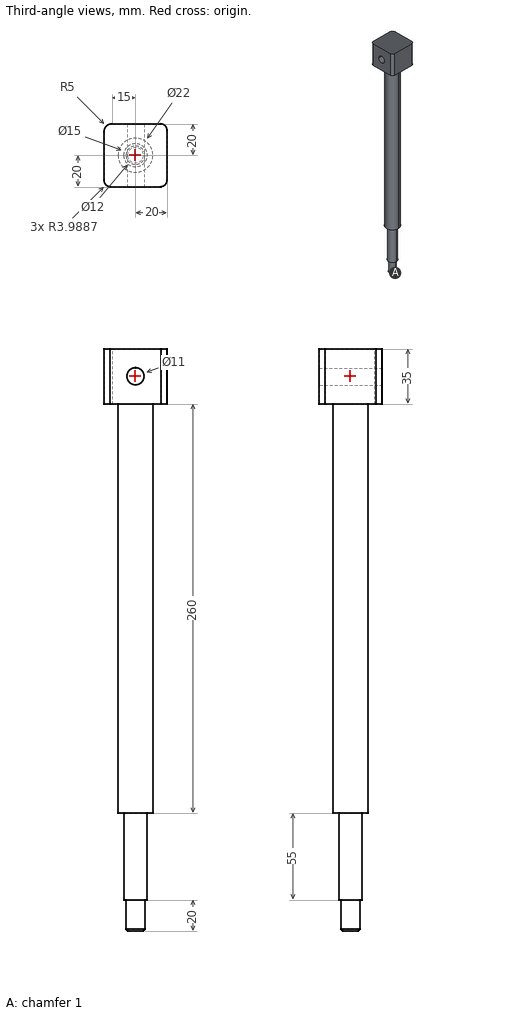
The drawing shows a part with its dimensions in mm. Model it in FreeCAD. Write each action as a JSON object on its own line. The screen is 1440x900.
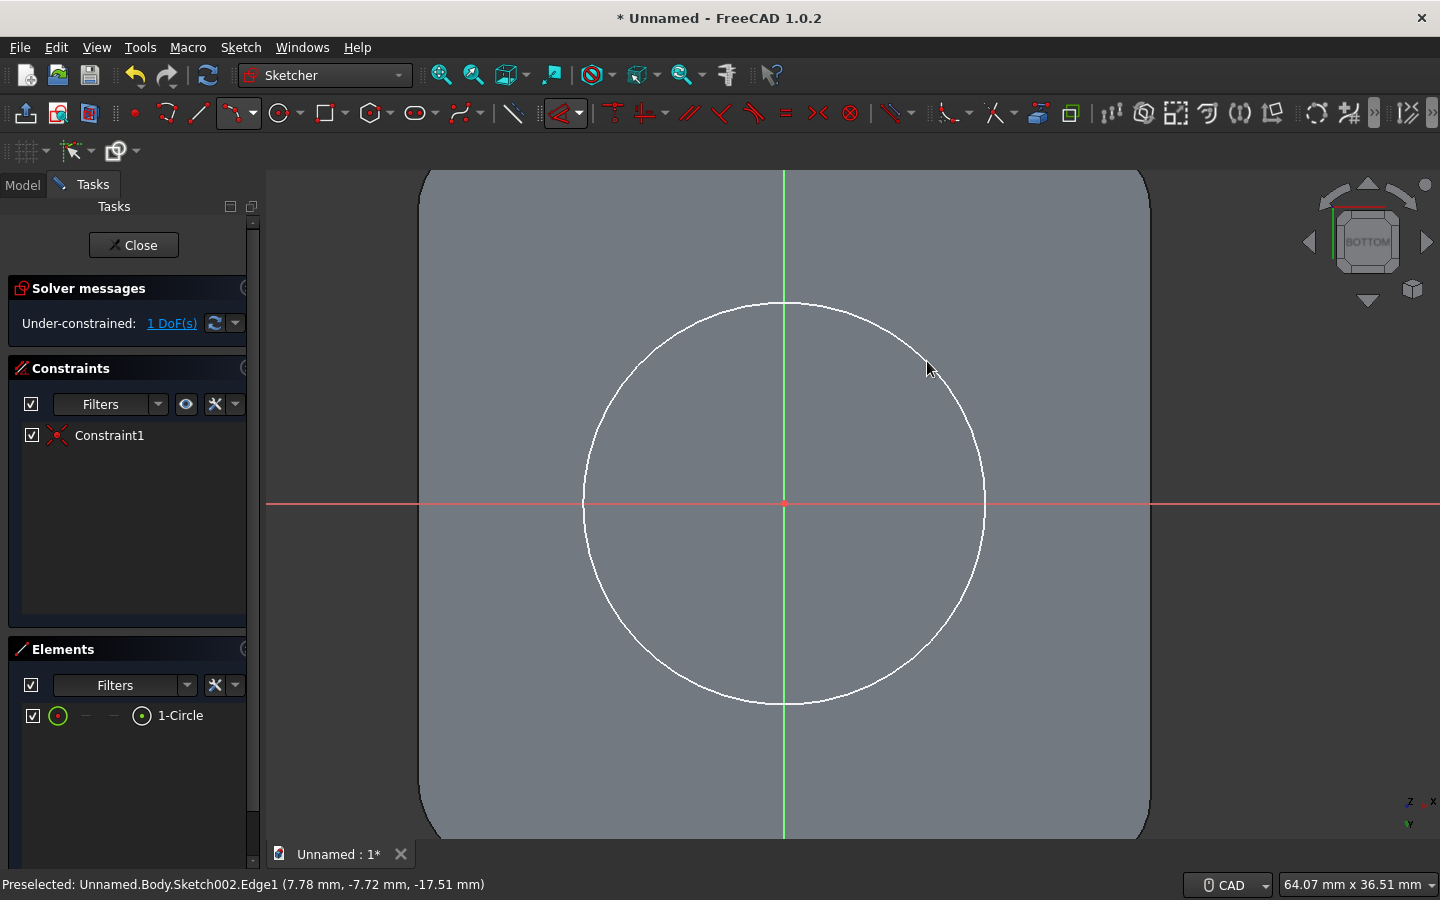
{"action": "left_click", "coordinate": [926, 361]}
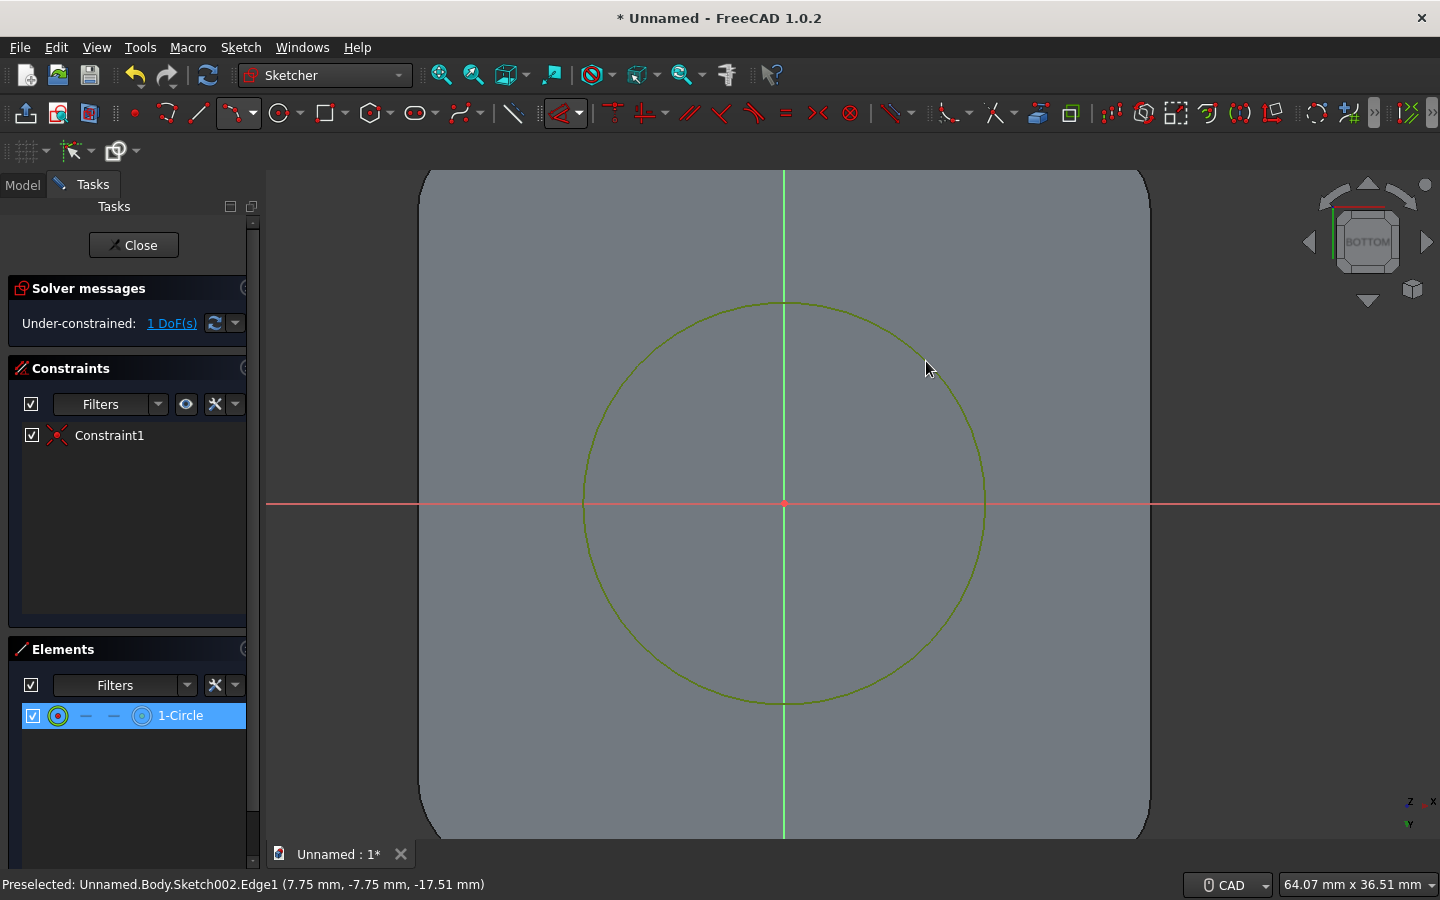
{"action": "left_click", "coordinate": [582, 114]}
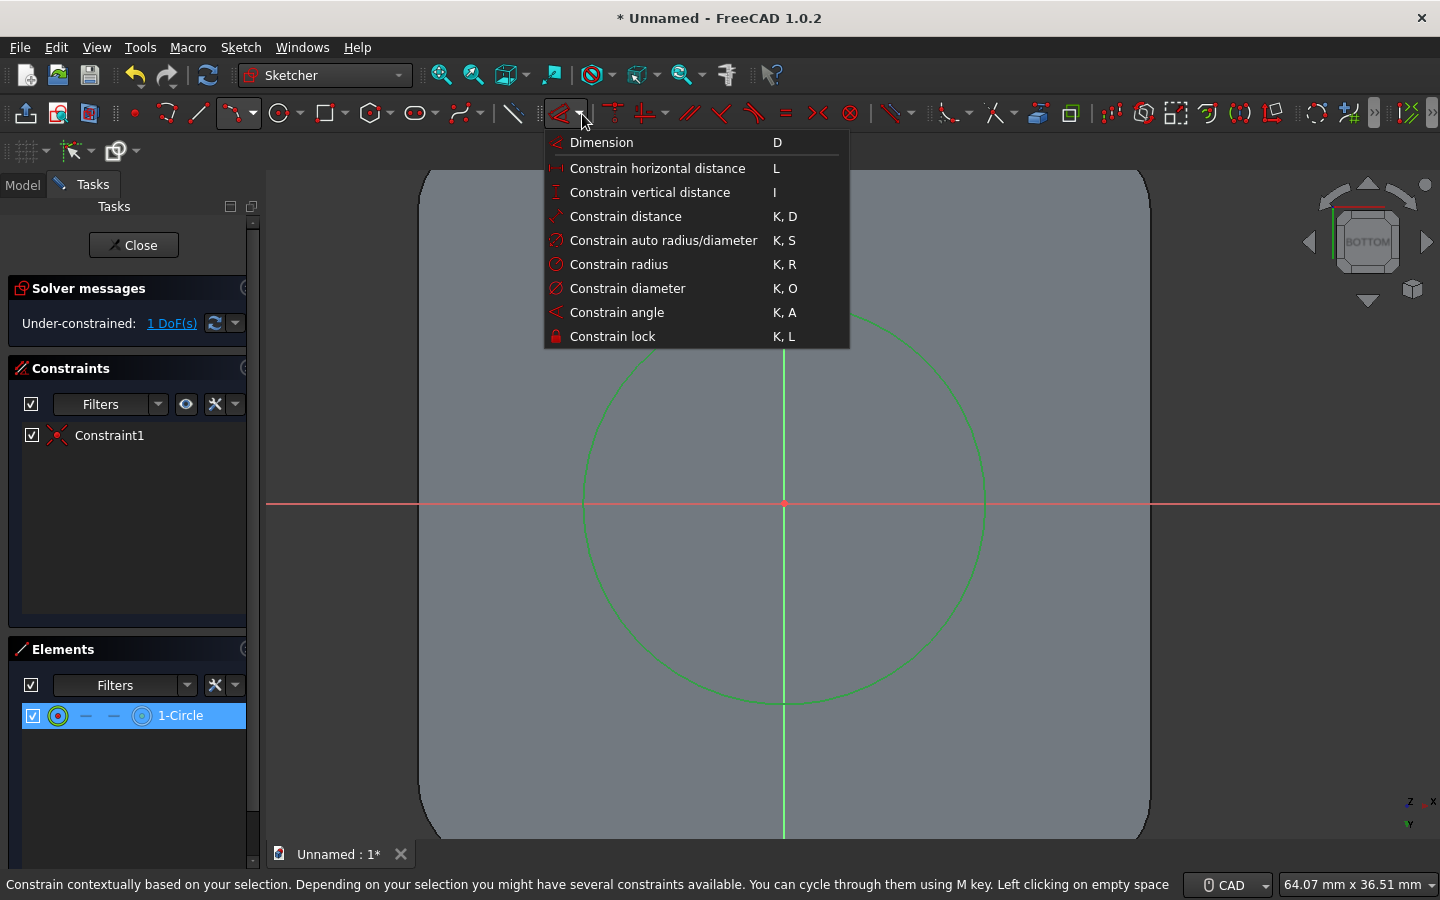
{"action": "left_click", "coordinate": [697, 288]}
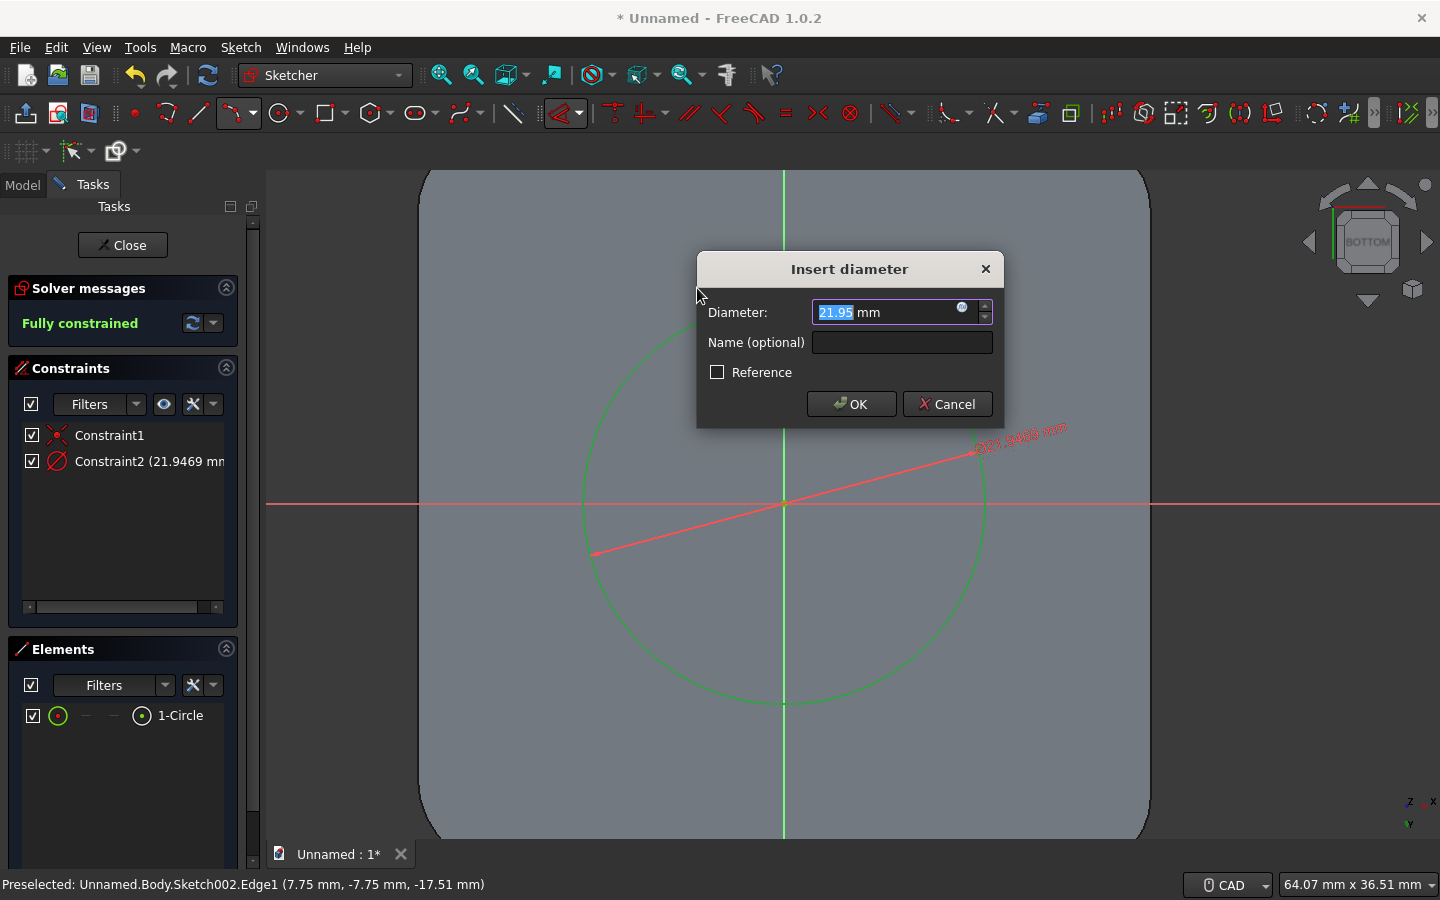
{"action": "type", "text": "22"}
{"action": "key", "text": "Return"}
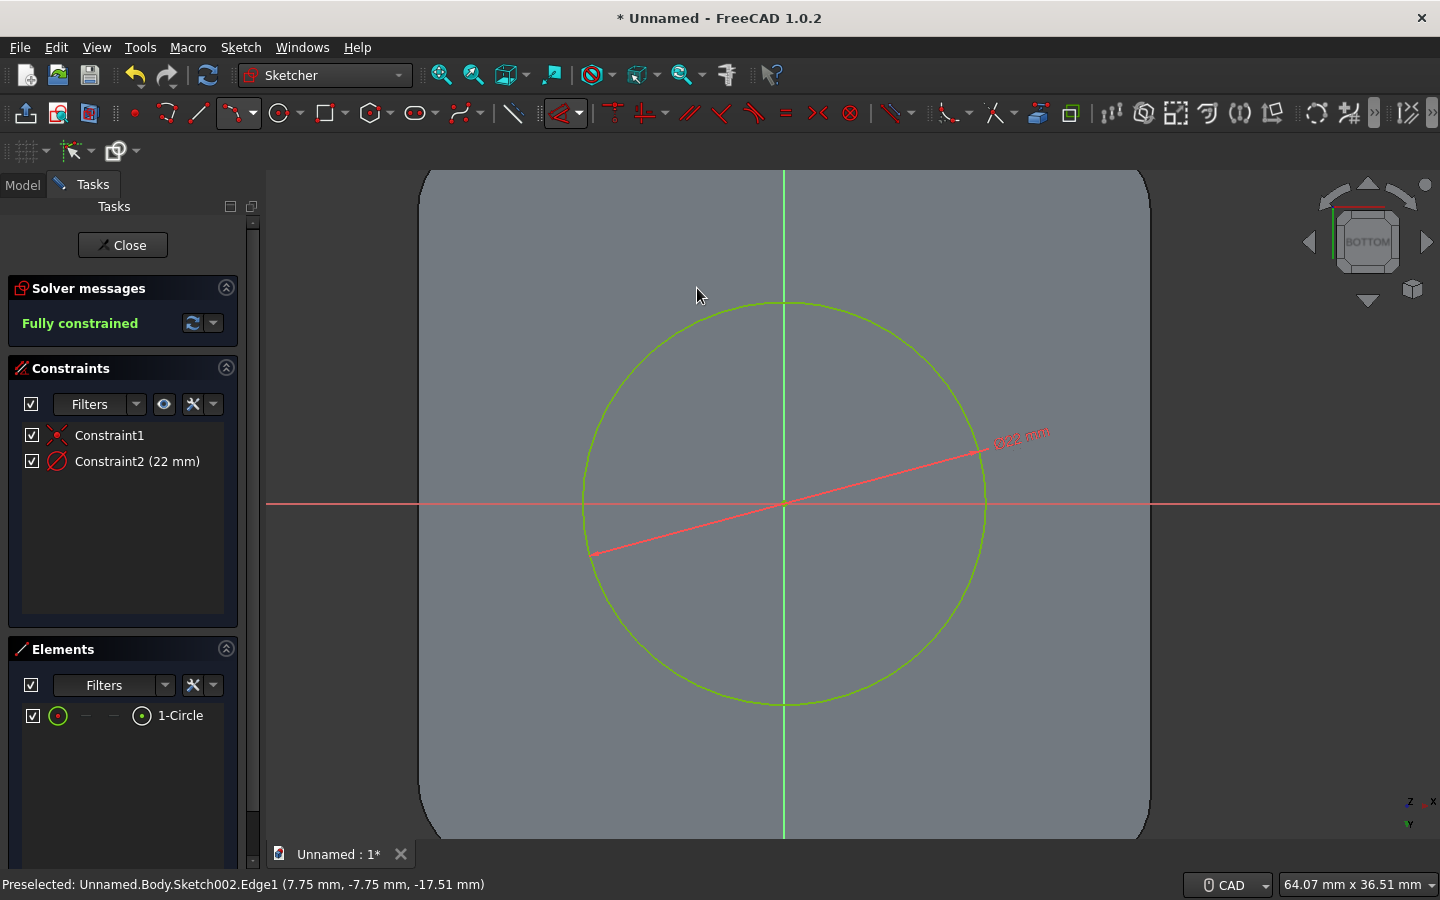
{"action": "left_click", "coordinate": [123, 245]}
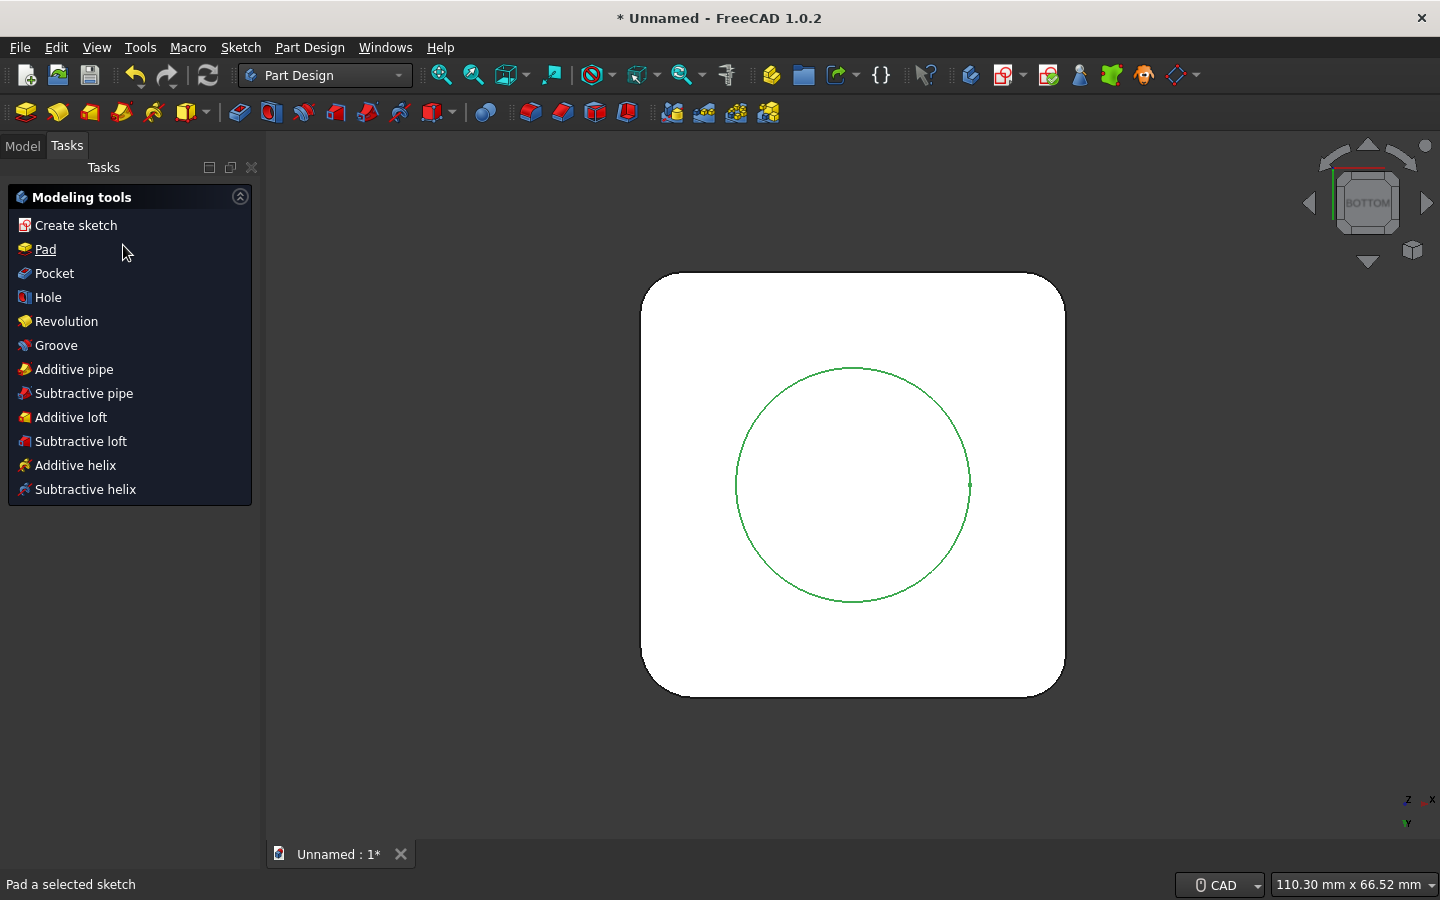
{"action": "left_click", "coordinate": [26, 112]}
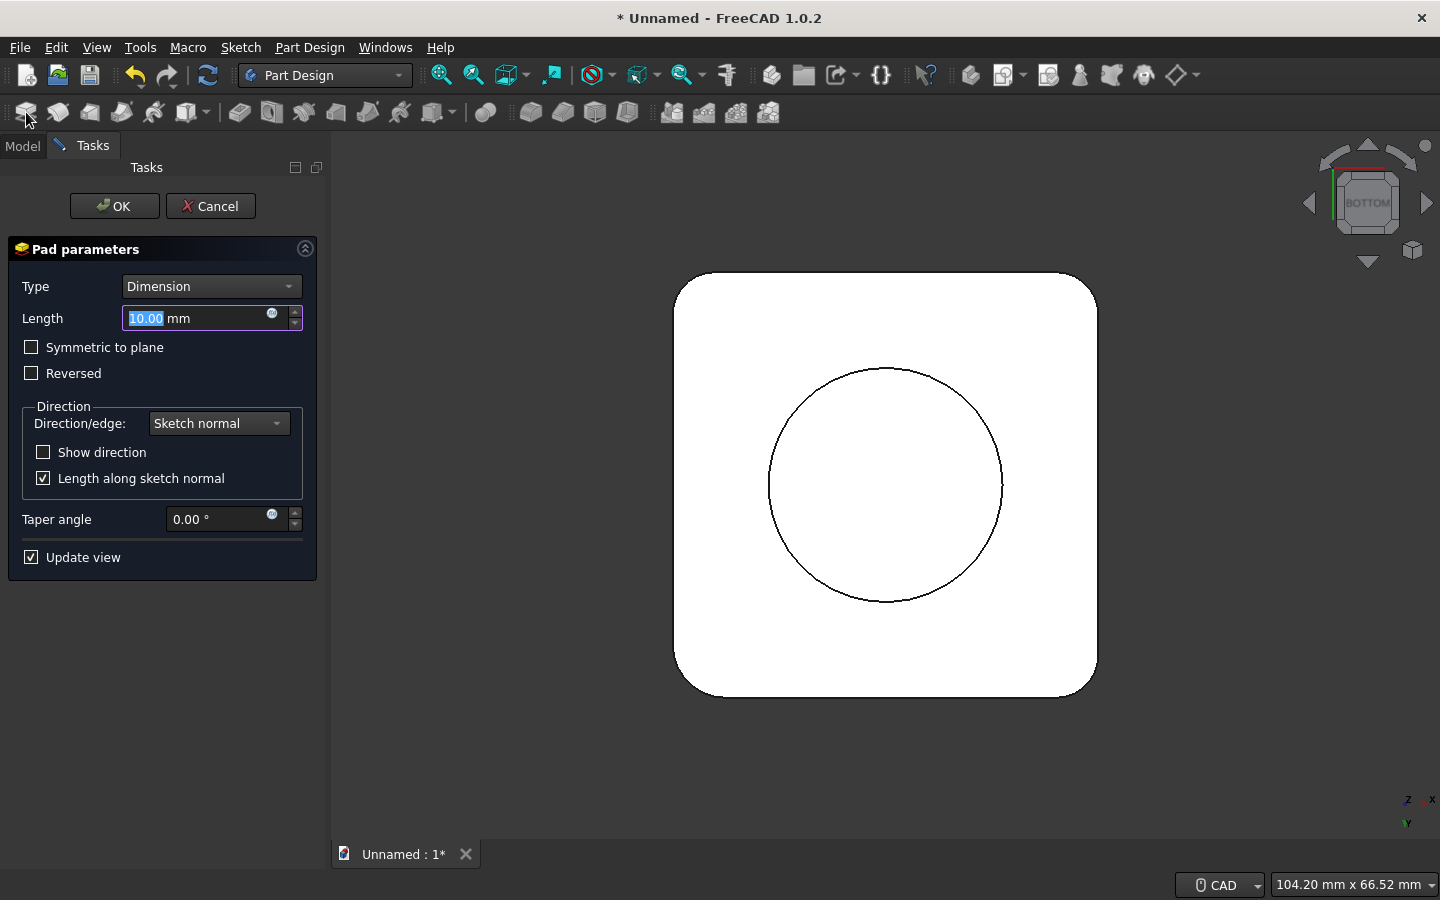
{"action": "type", "text": "260"}
{"action": "key", "text": "Tab"}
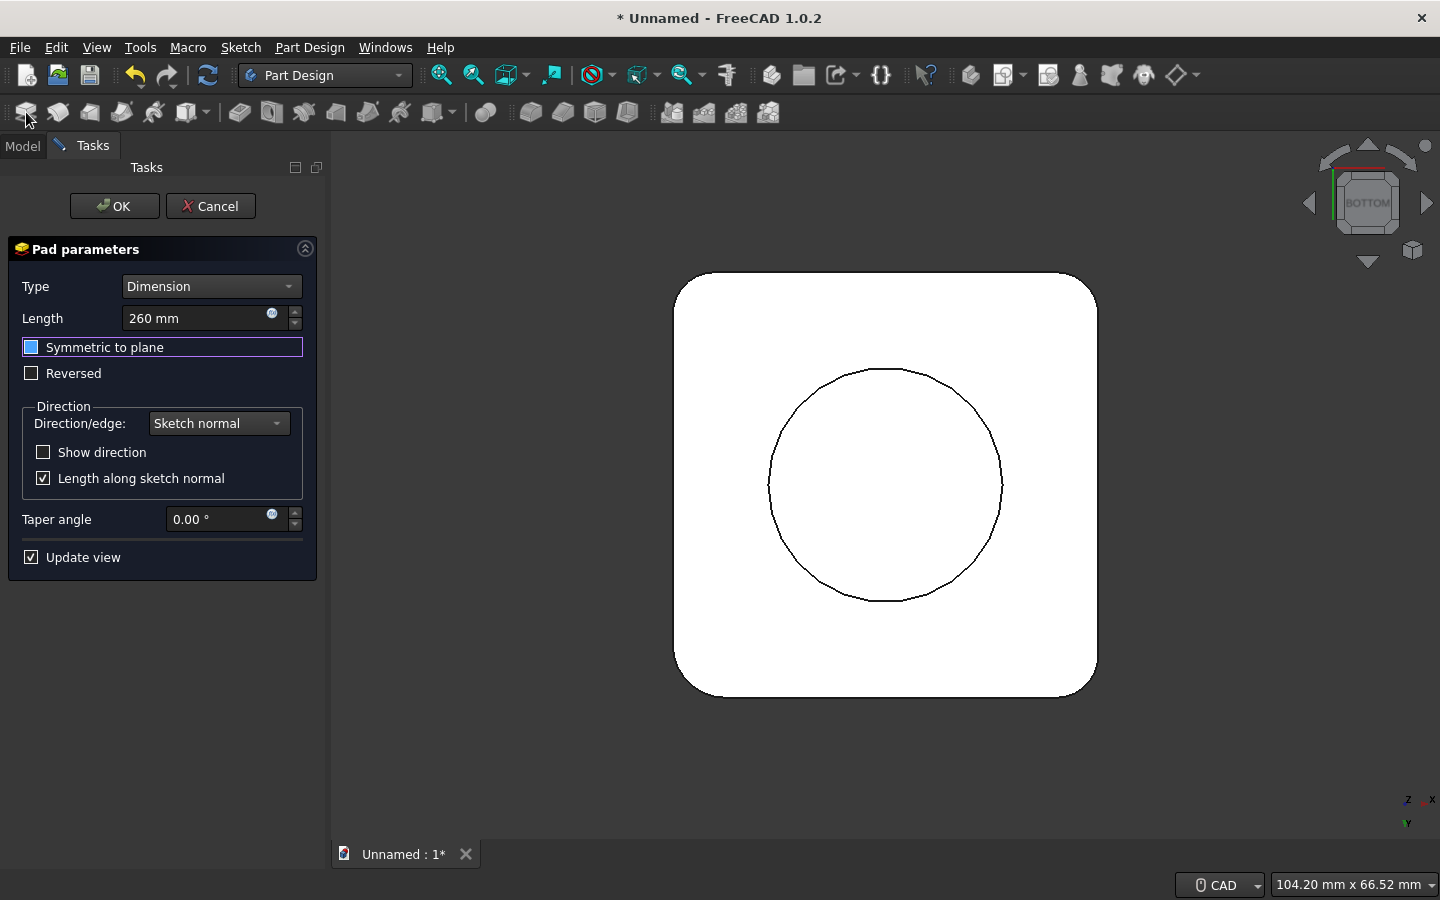
{"action": "left_click", "coordinate": [115, 206]}